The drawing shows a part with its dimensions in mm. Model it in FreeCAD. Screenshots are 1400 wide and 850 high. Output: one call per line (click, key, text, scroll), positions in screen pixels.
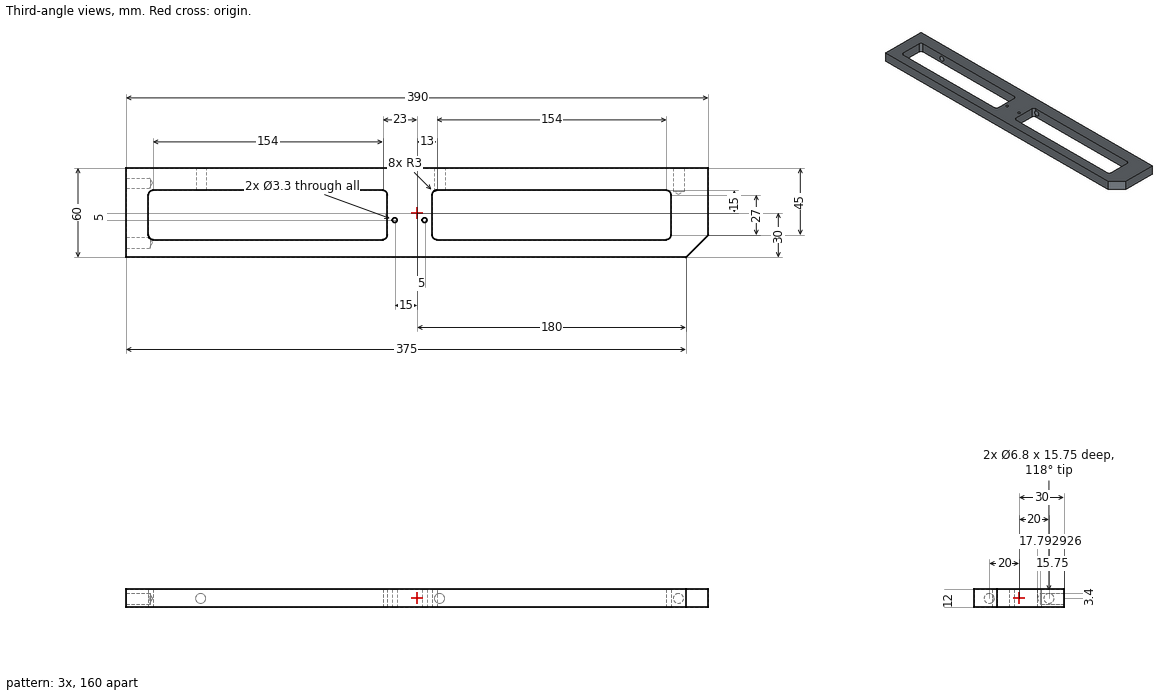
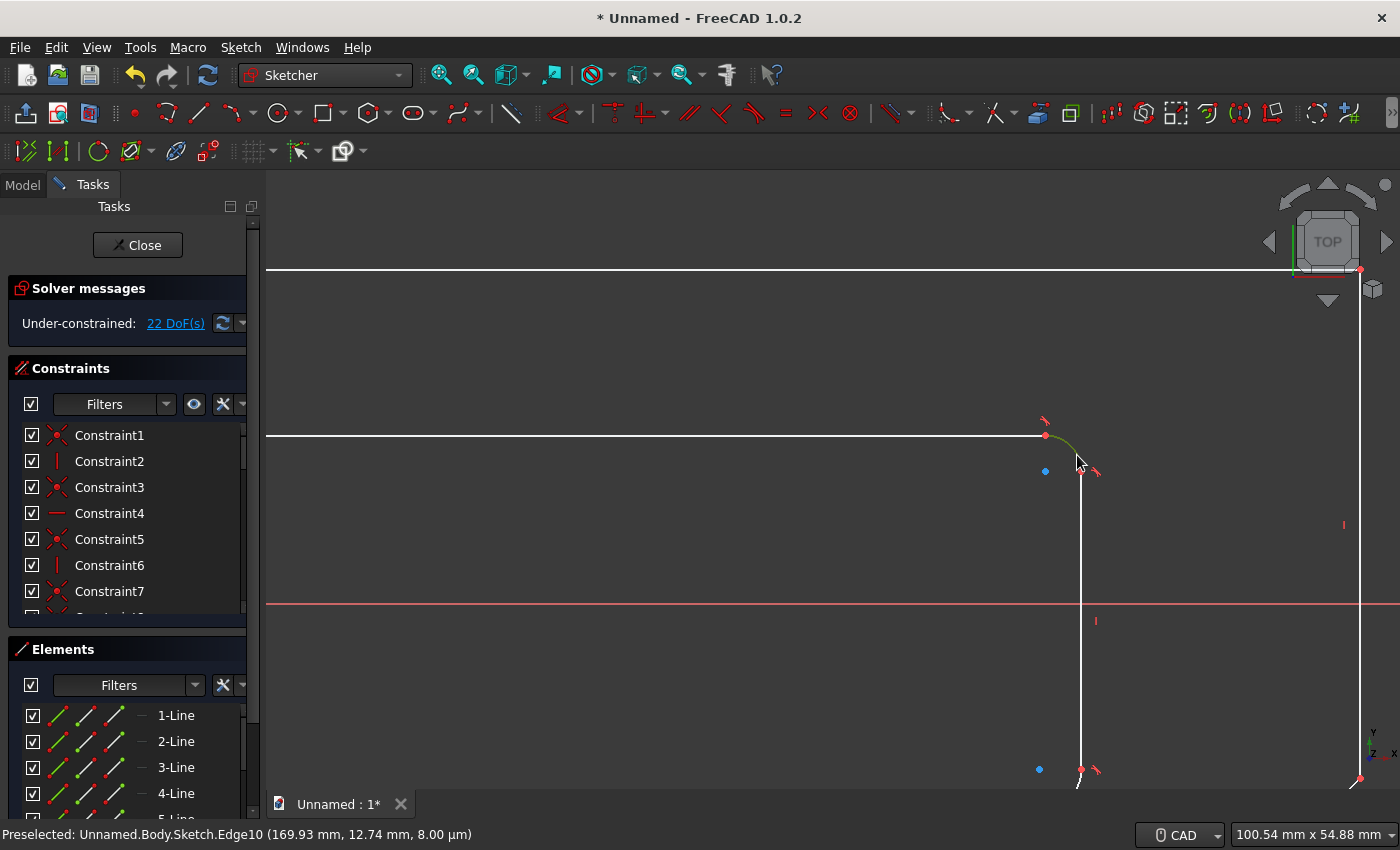
scroll(1082, 455, down, 9)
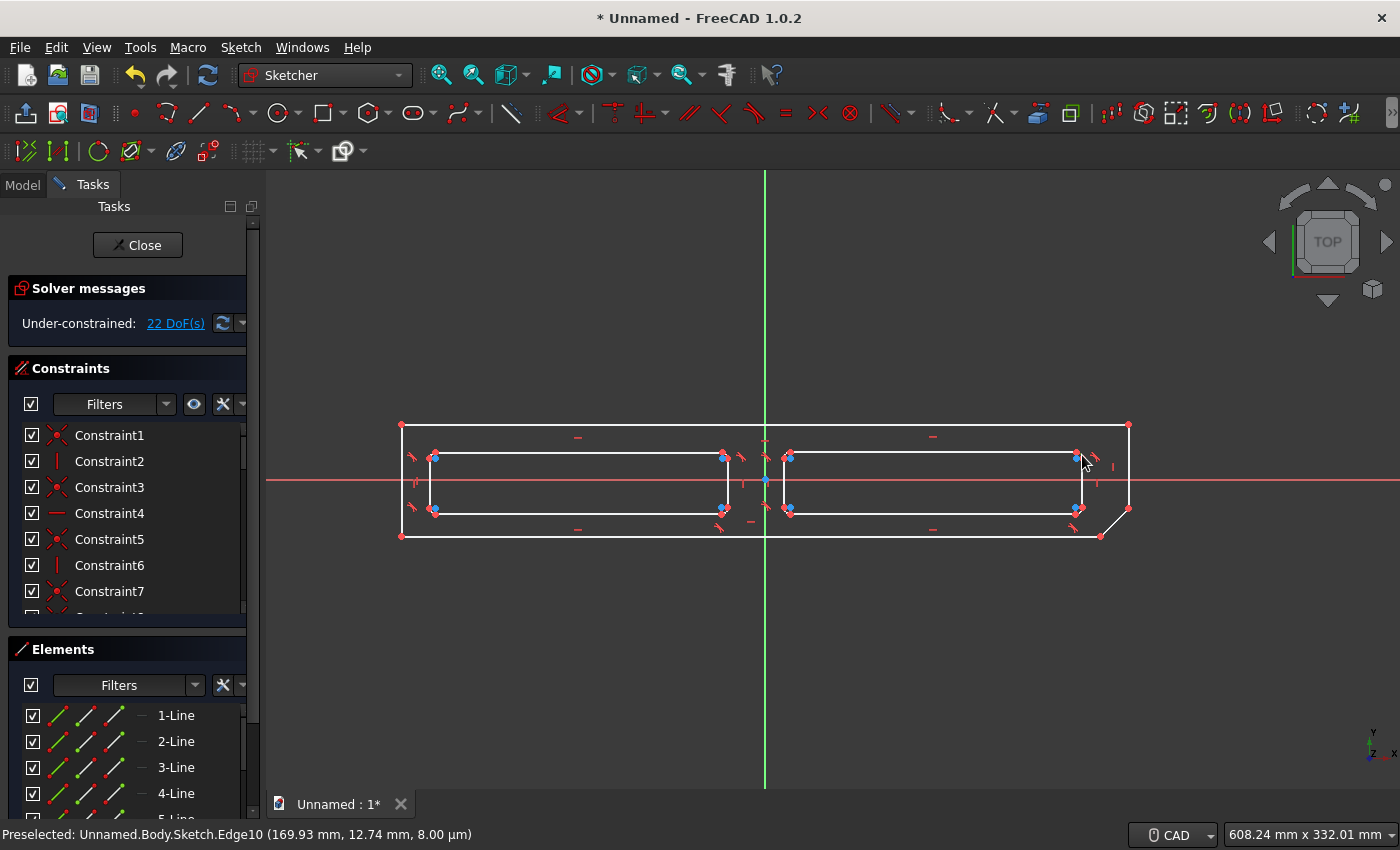
scroll(1079, 514, up, 8)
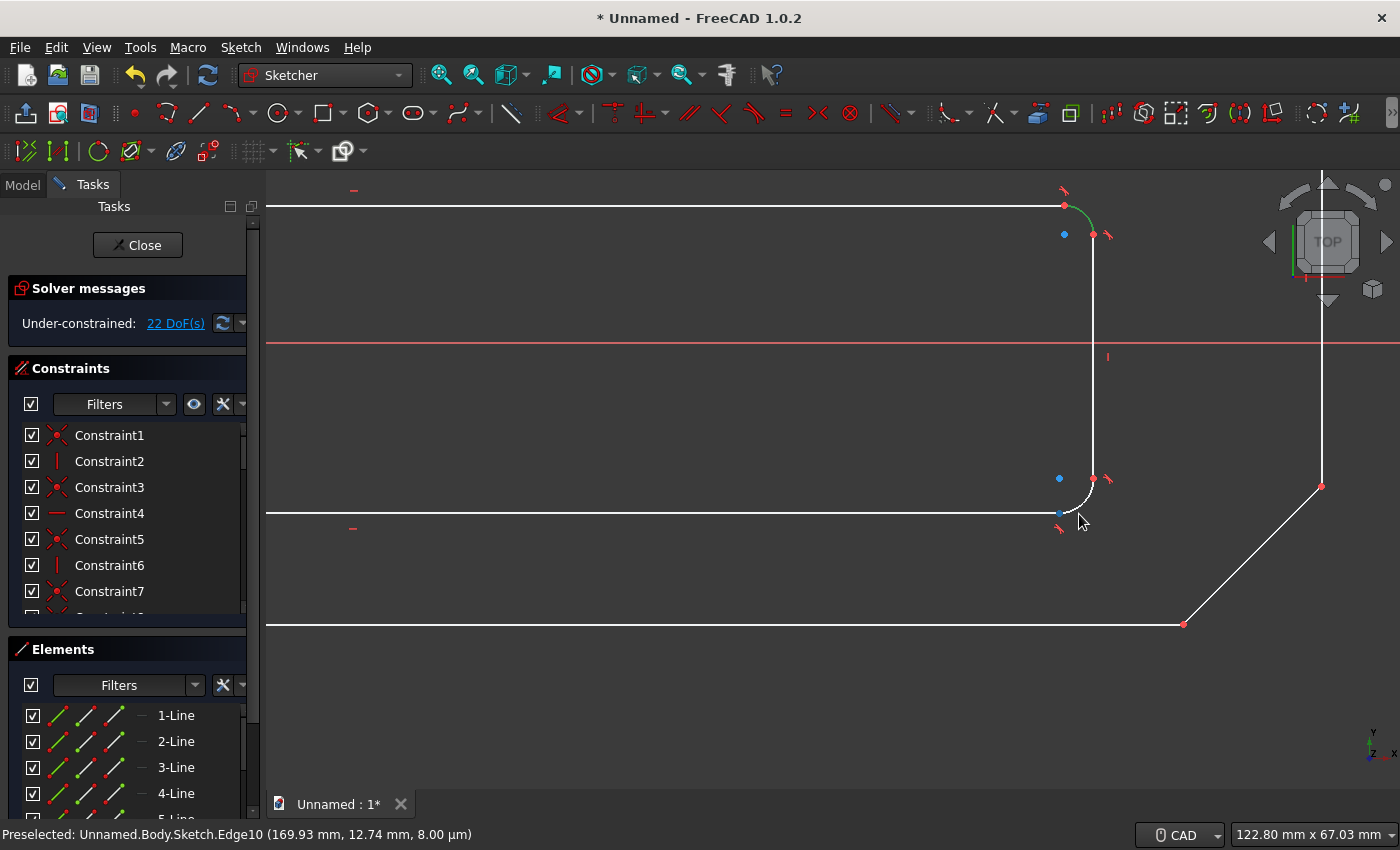
click(1075, 509)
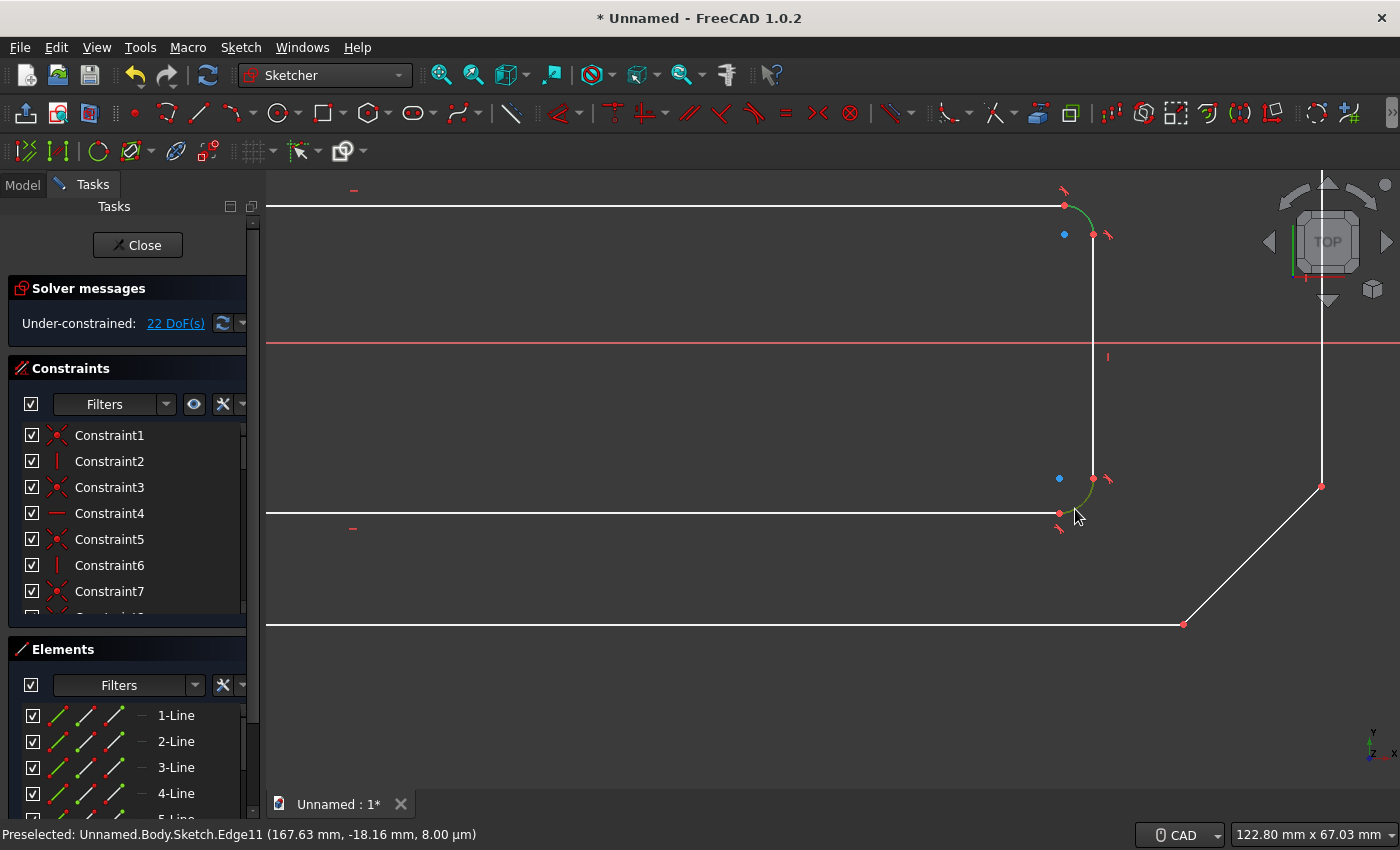
scroll(1079, 514, down, 8)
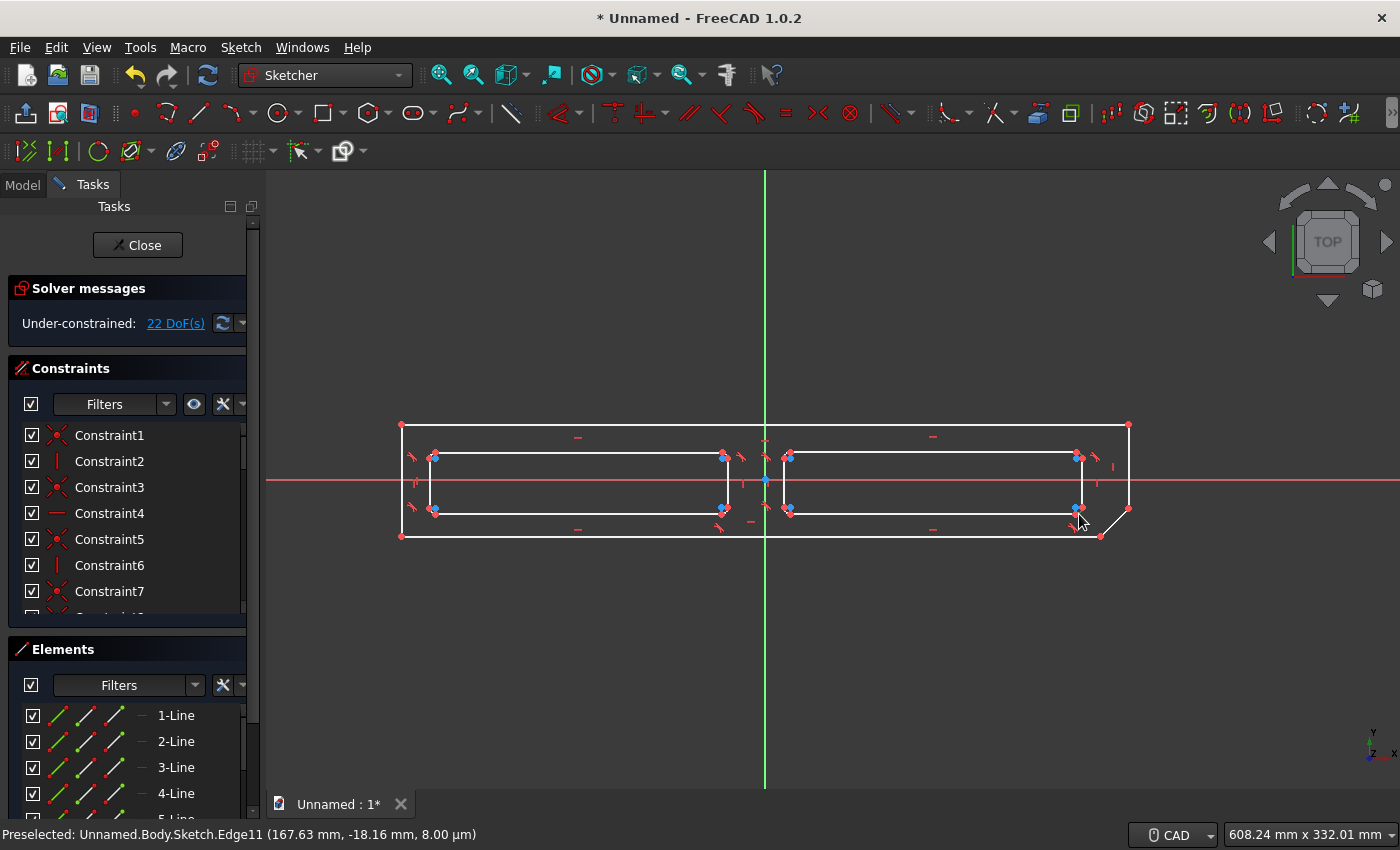
scroll(785, 511, up, 8)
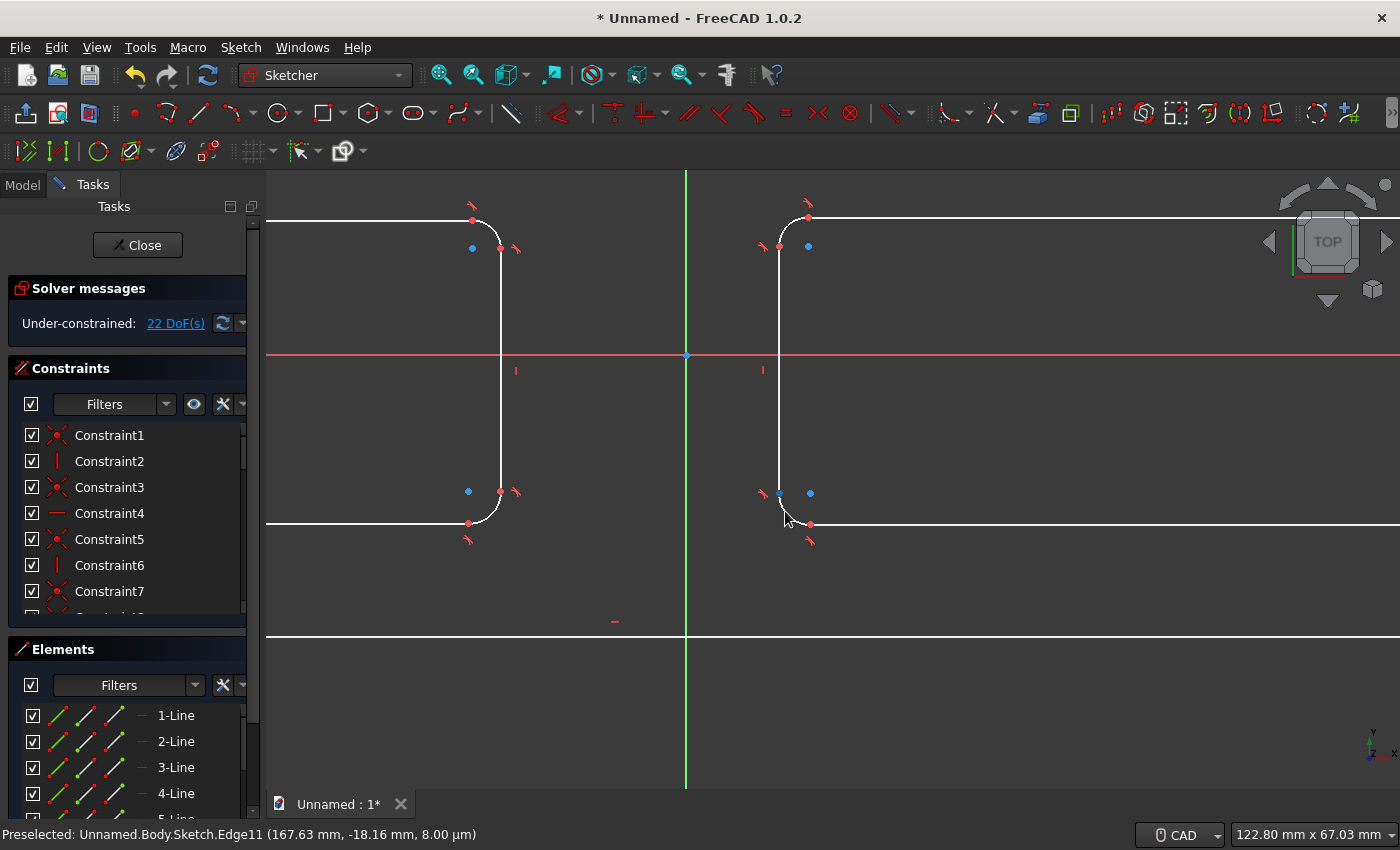
click(783, 508)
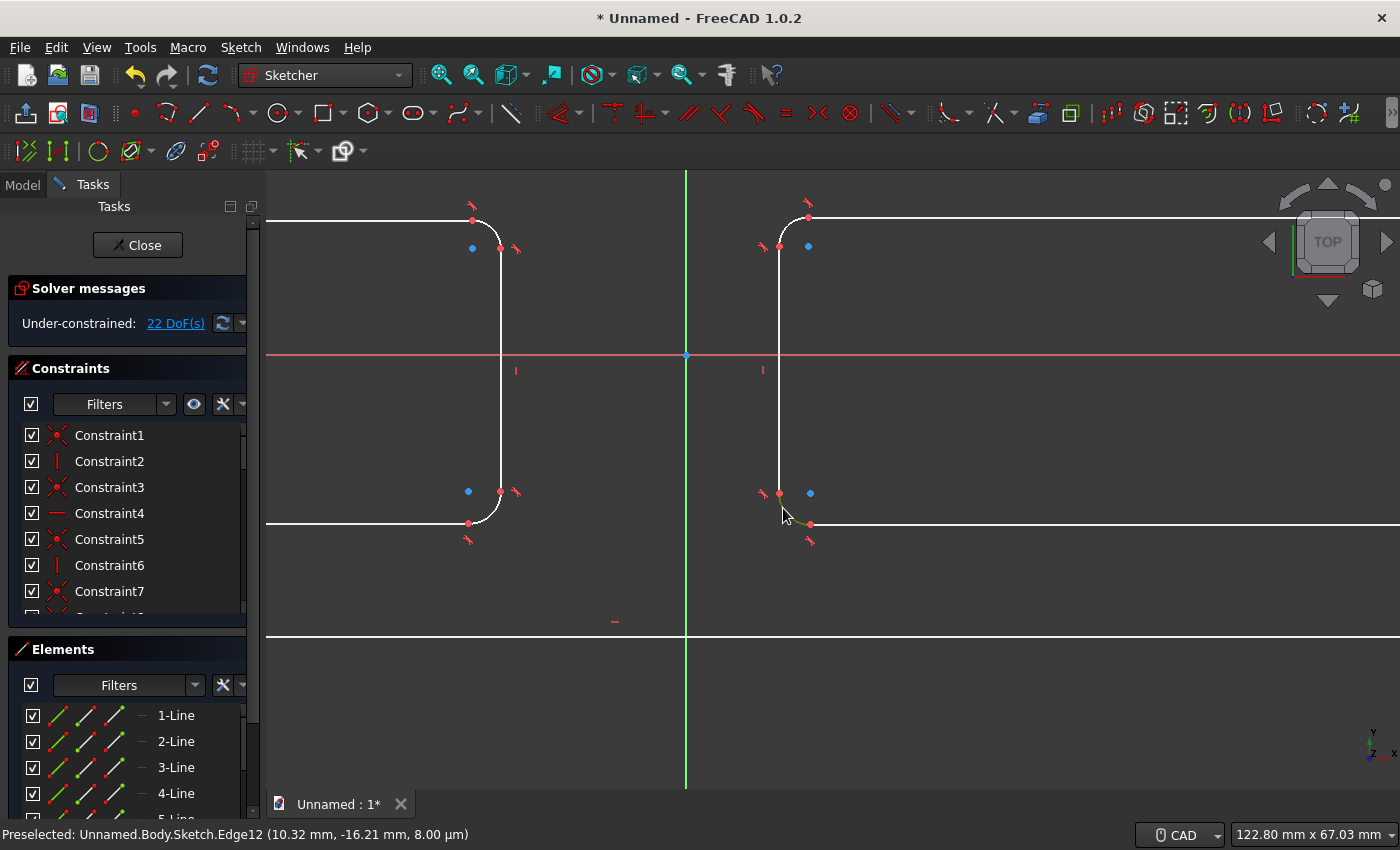
click(795, 221)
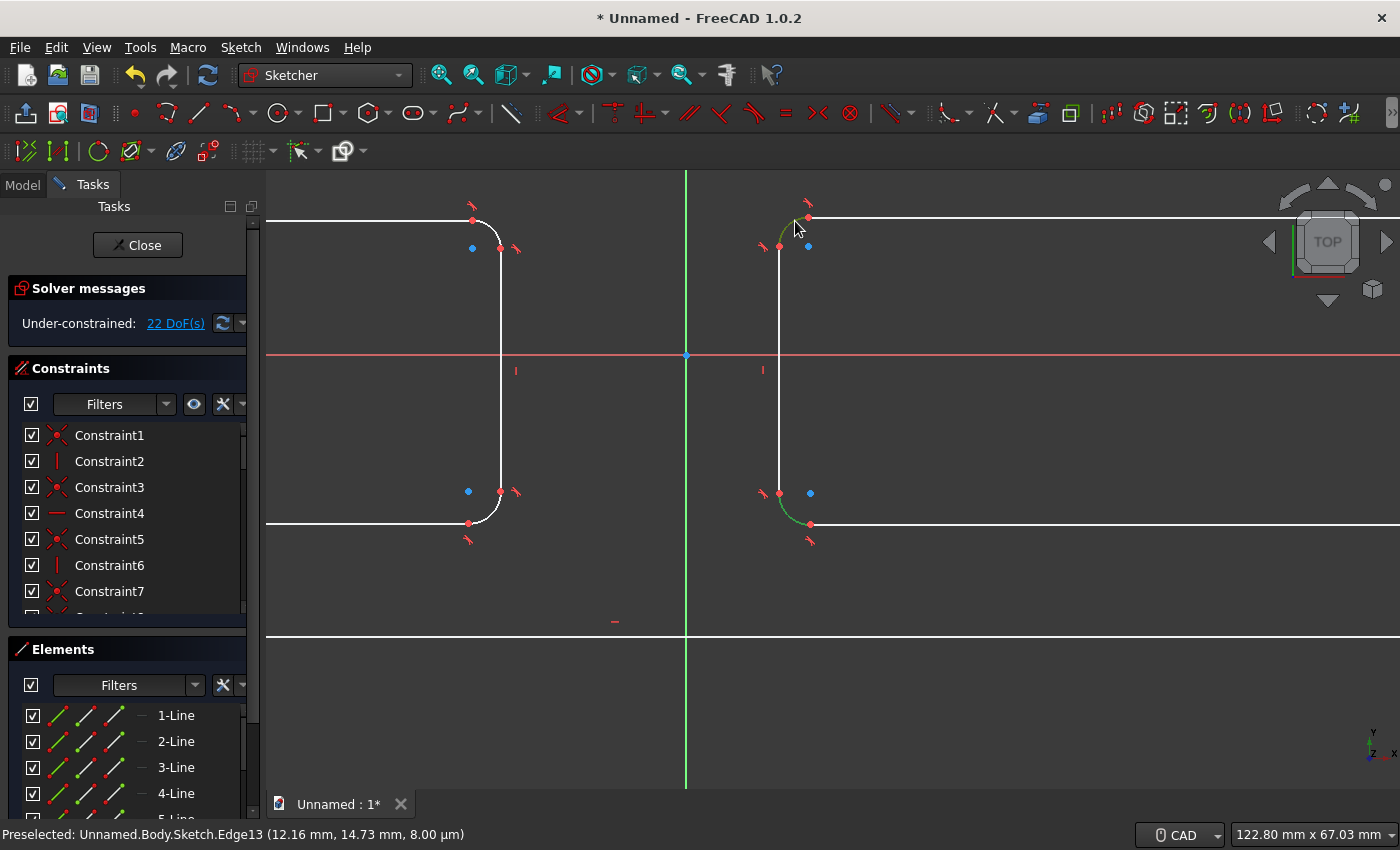
click(498, 236)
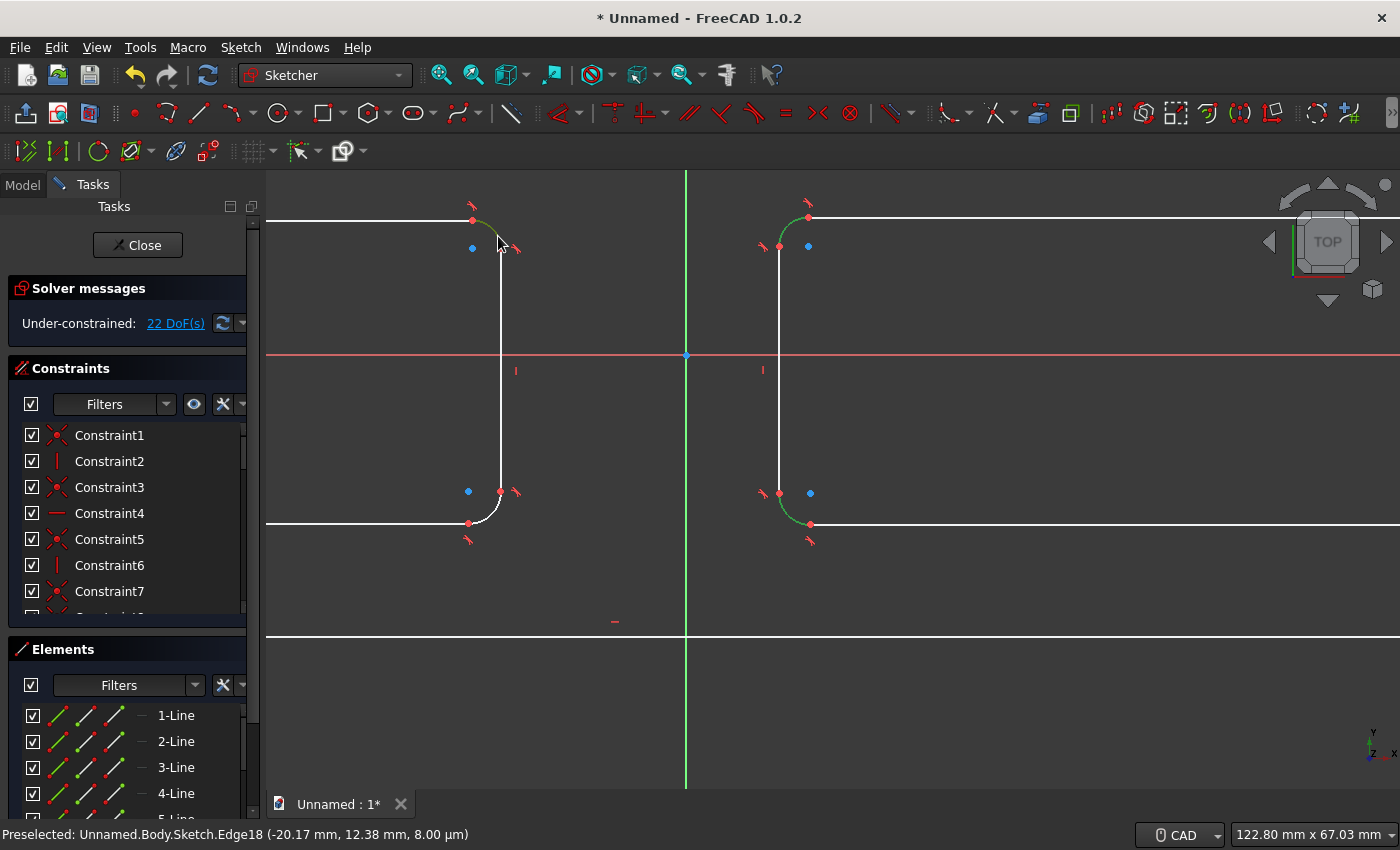
click(483, 520)